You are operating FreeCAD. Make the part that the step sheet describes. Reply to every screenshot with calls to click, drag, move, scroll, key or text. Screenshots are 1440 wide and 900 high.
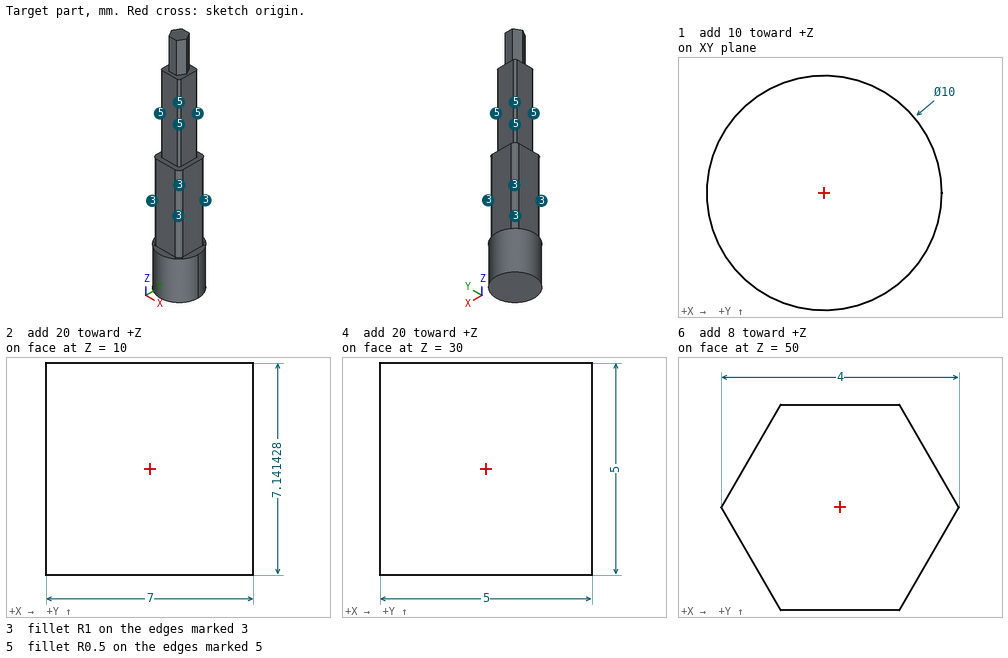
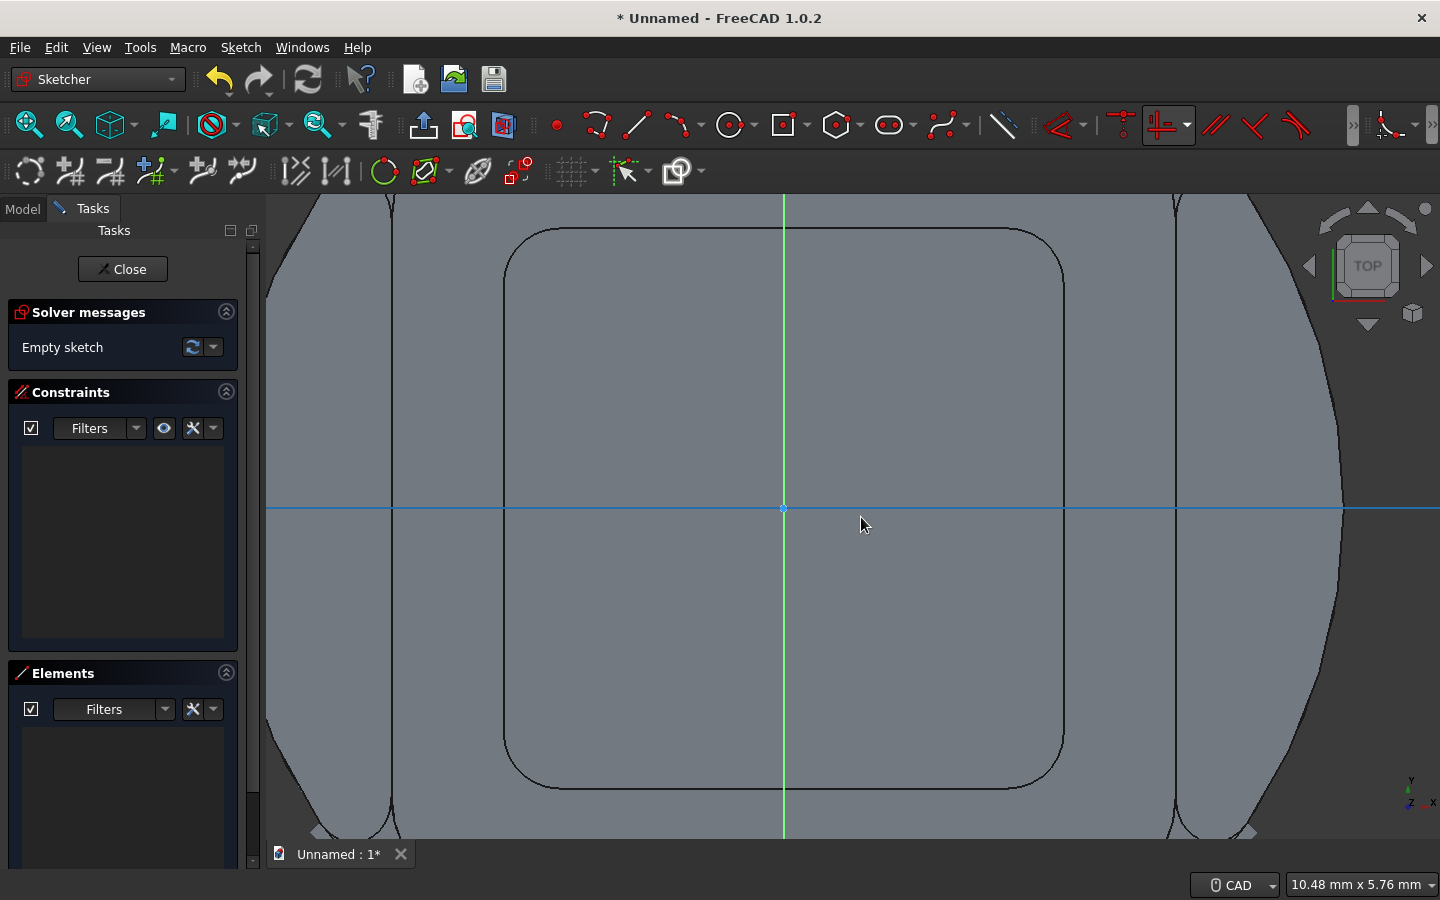
click(836, 126)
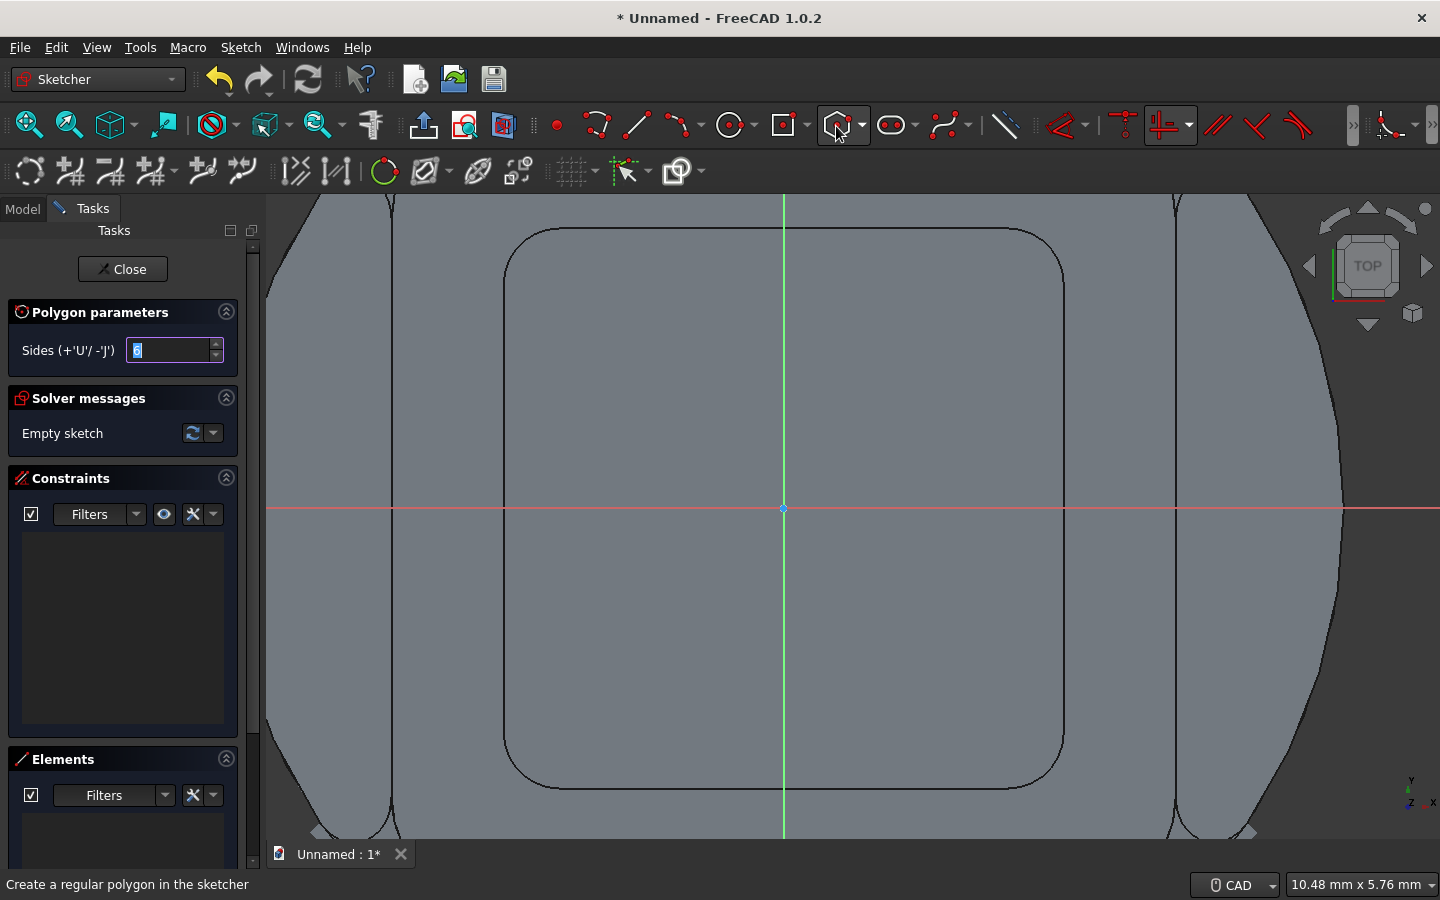
click(784, 508)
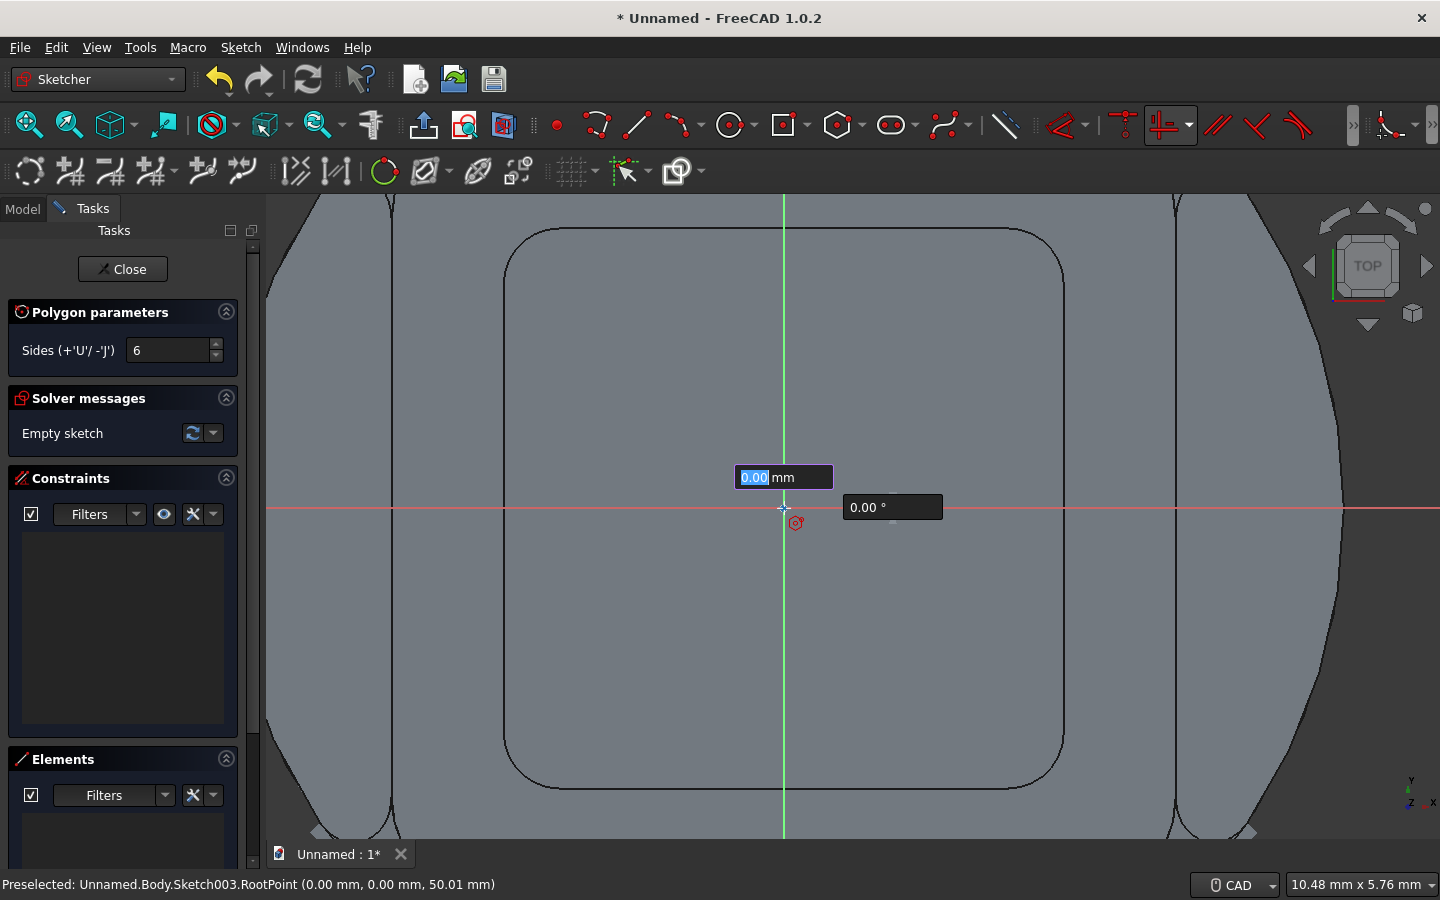
click(560, 508)
key(Escape)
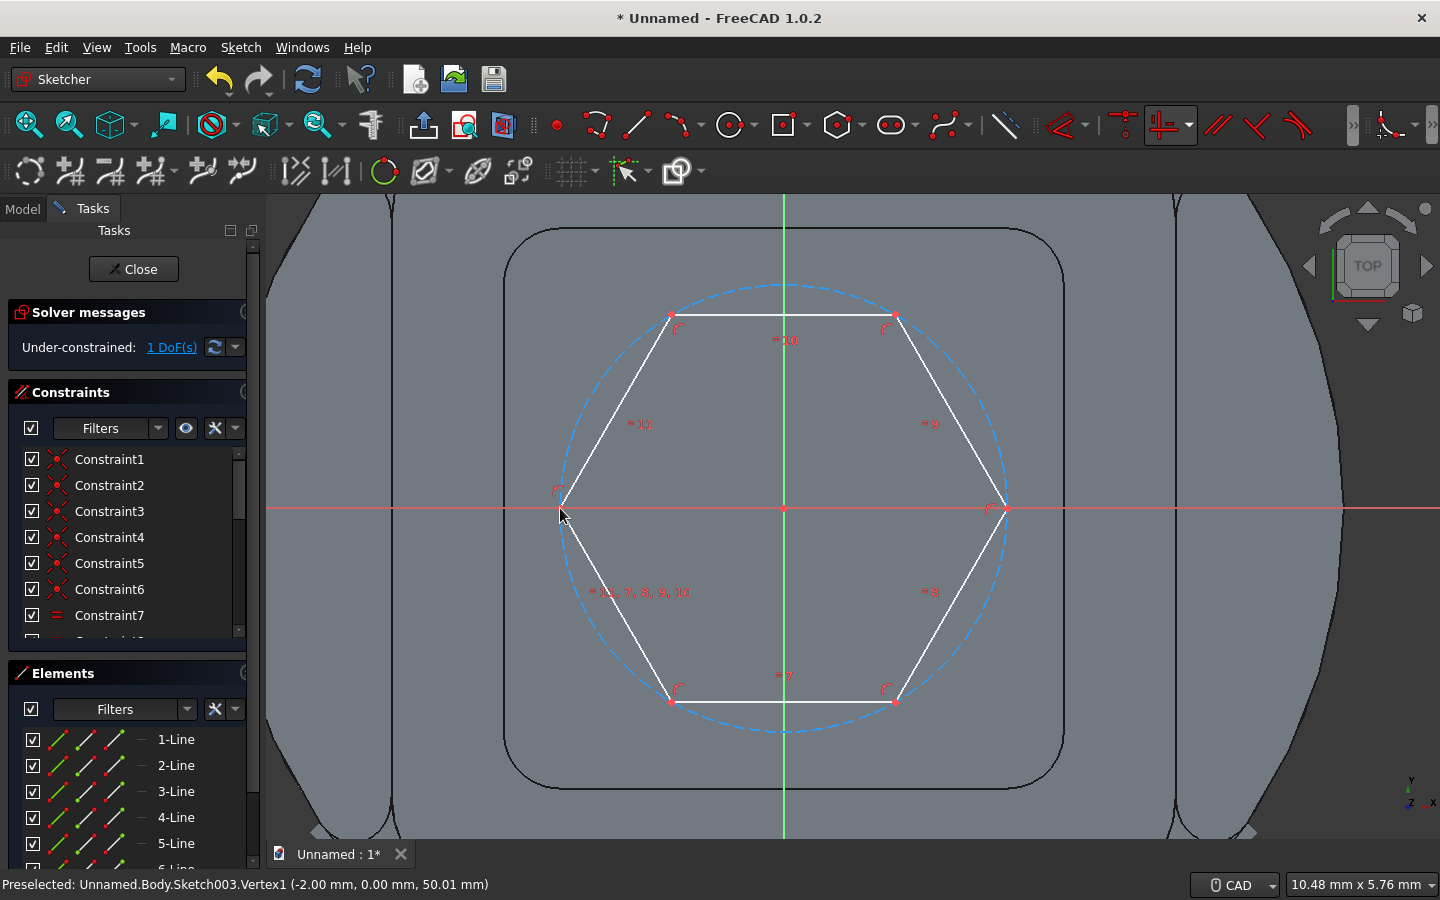
click(1060, 126)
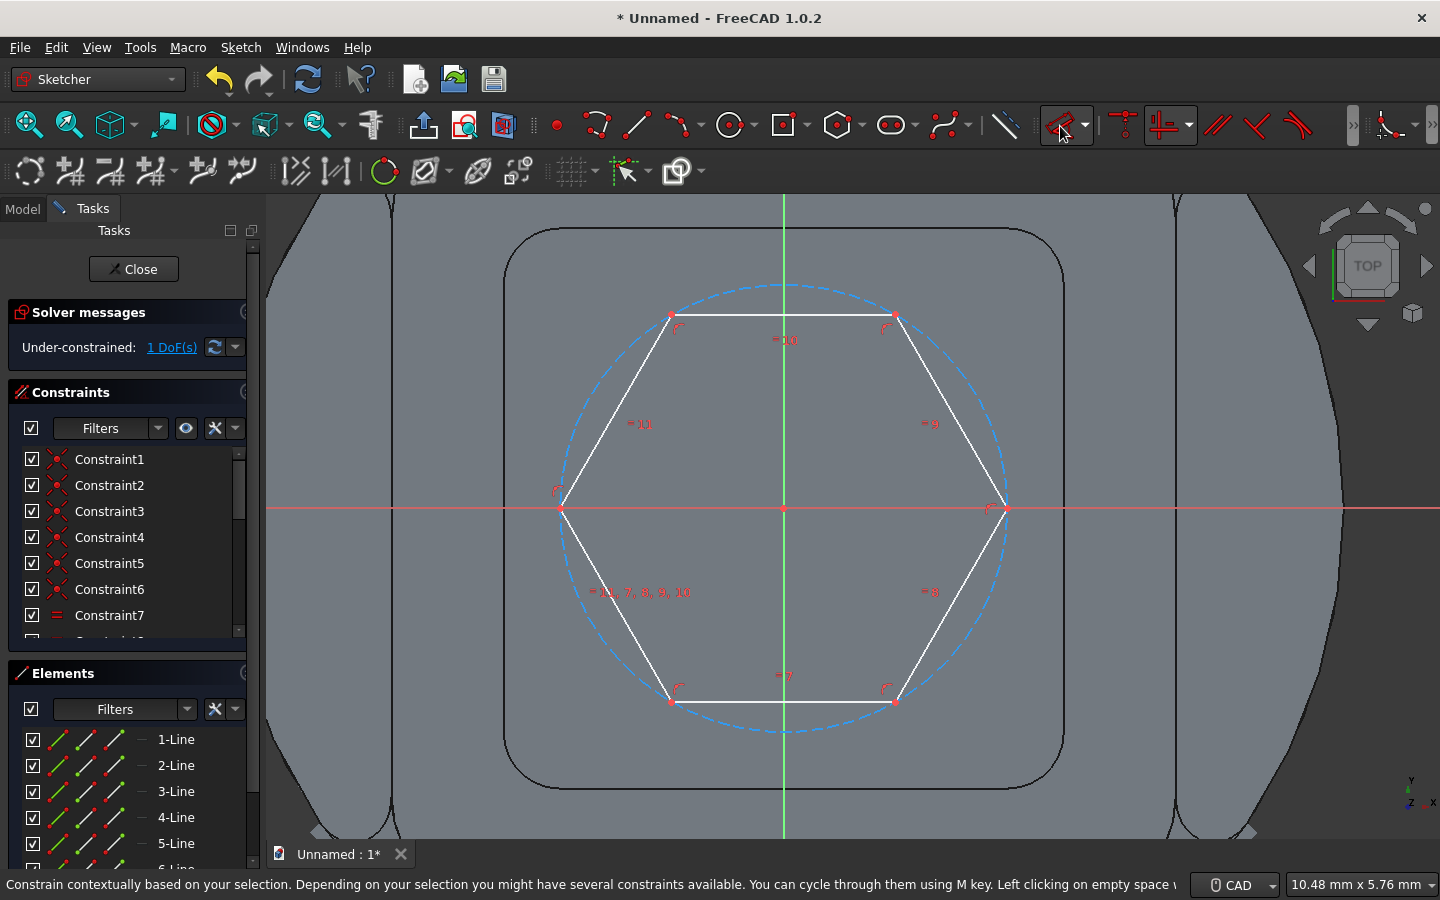
click(560, 508)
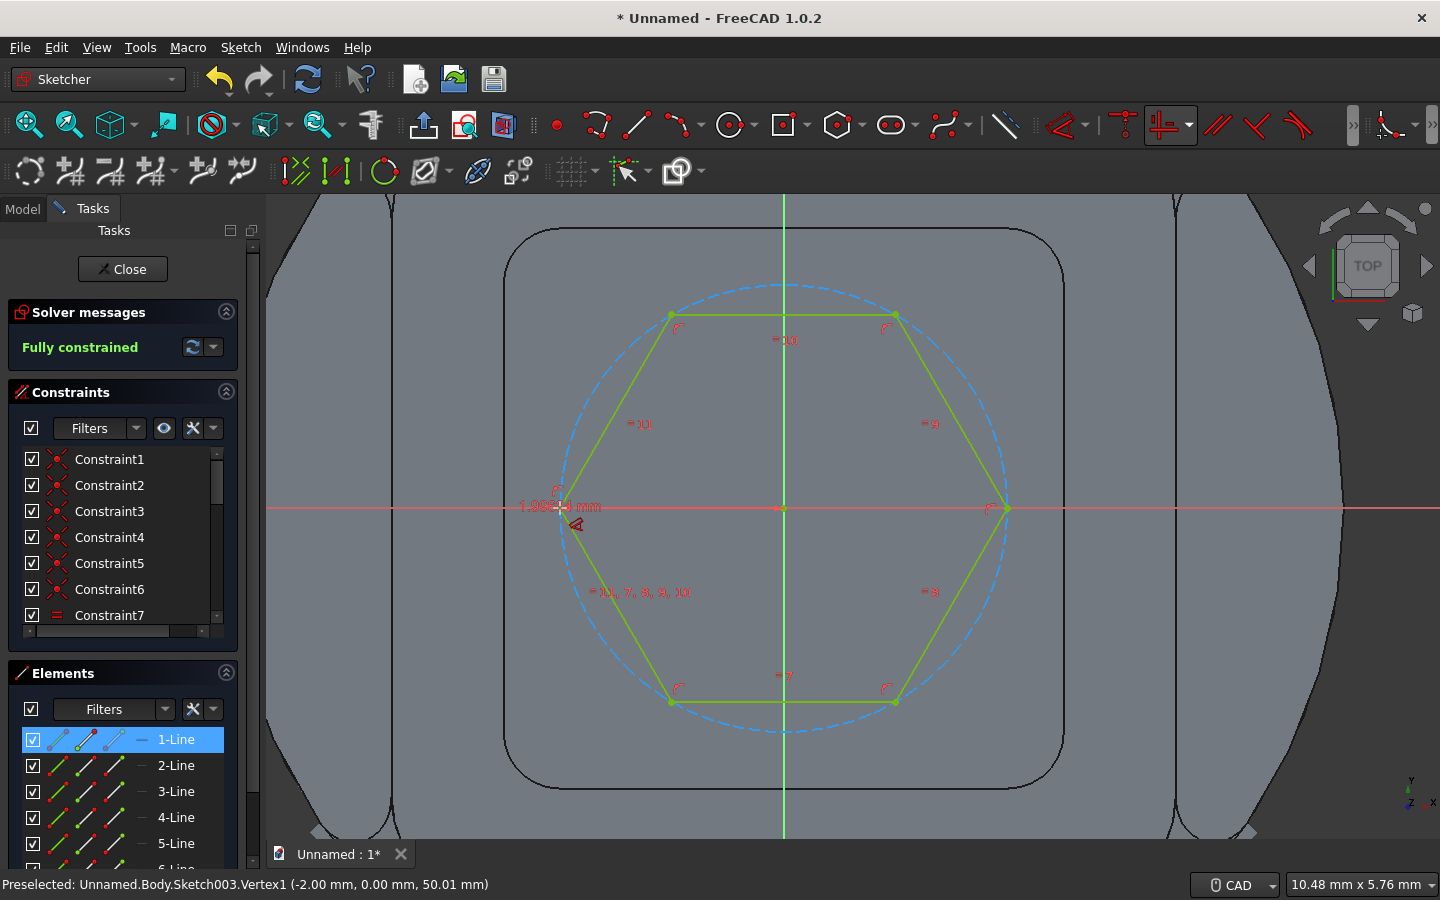
click(1007, 508)
click(681, 542)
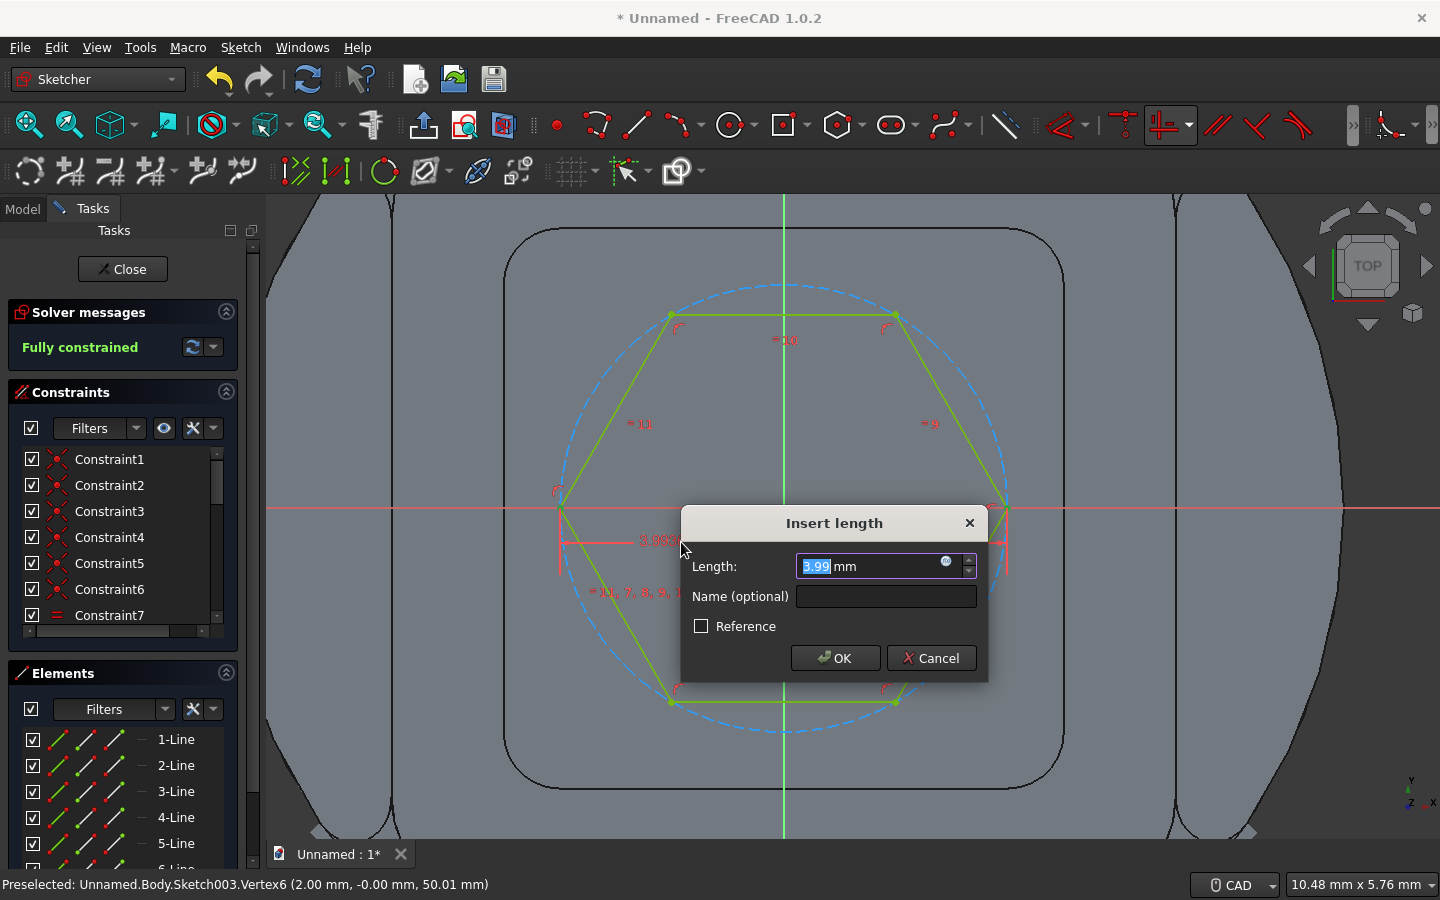
text(4)
key(Return)
key(Escape)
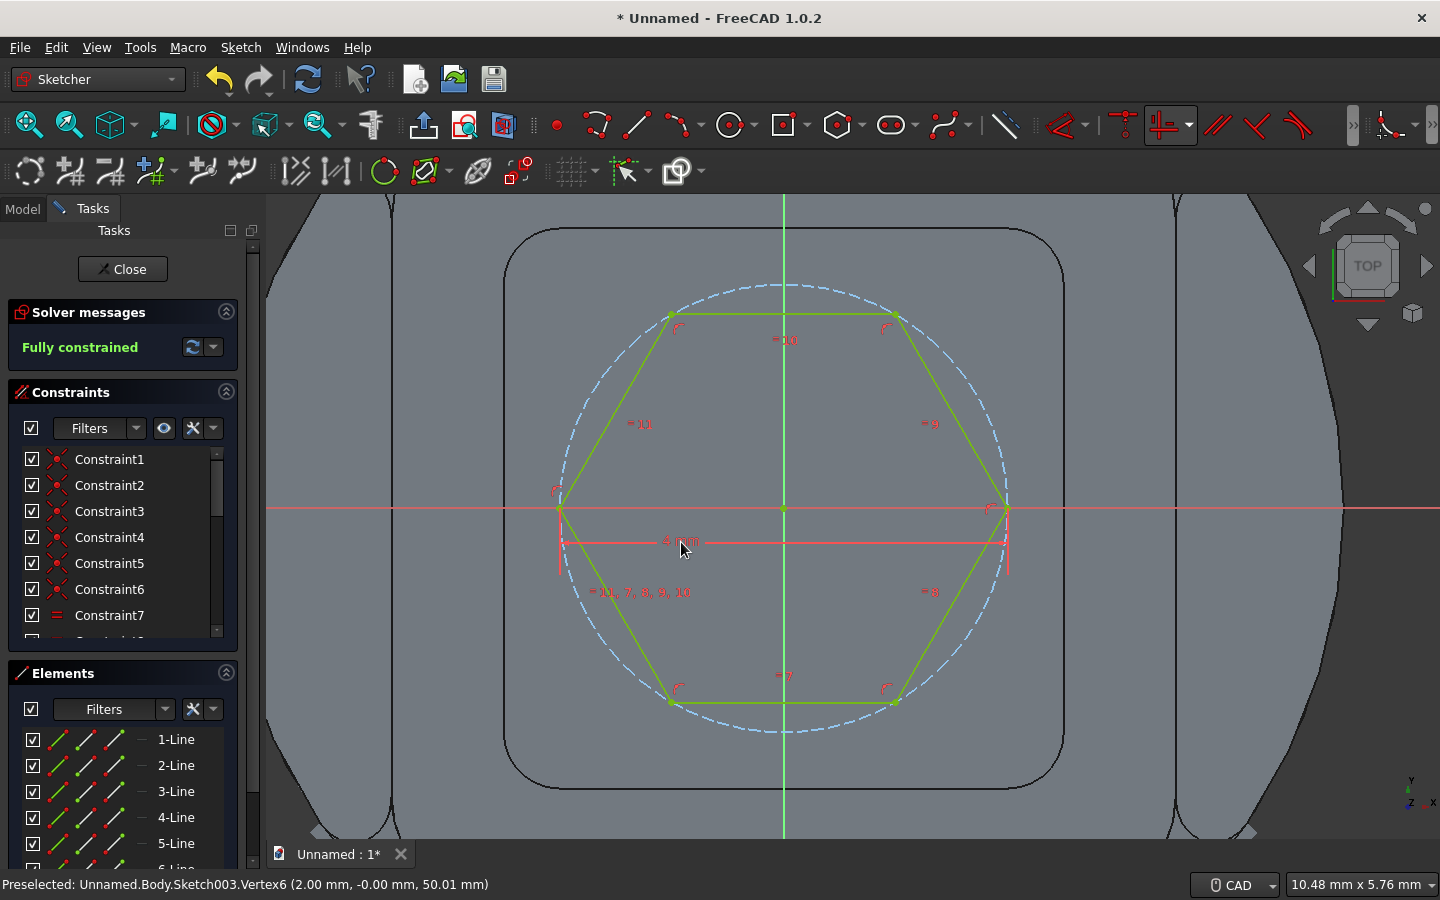
click(123, 269)